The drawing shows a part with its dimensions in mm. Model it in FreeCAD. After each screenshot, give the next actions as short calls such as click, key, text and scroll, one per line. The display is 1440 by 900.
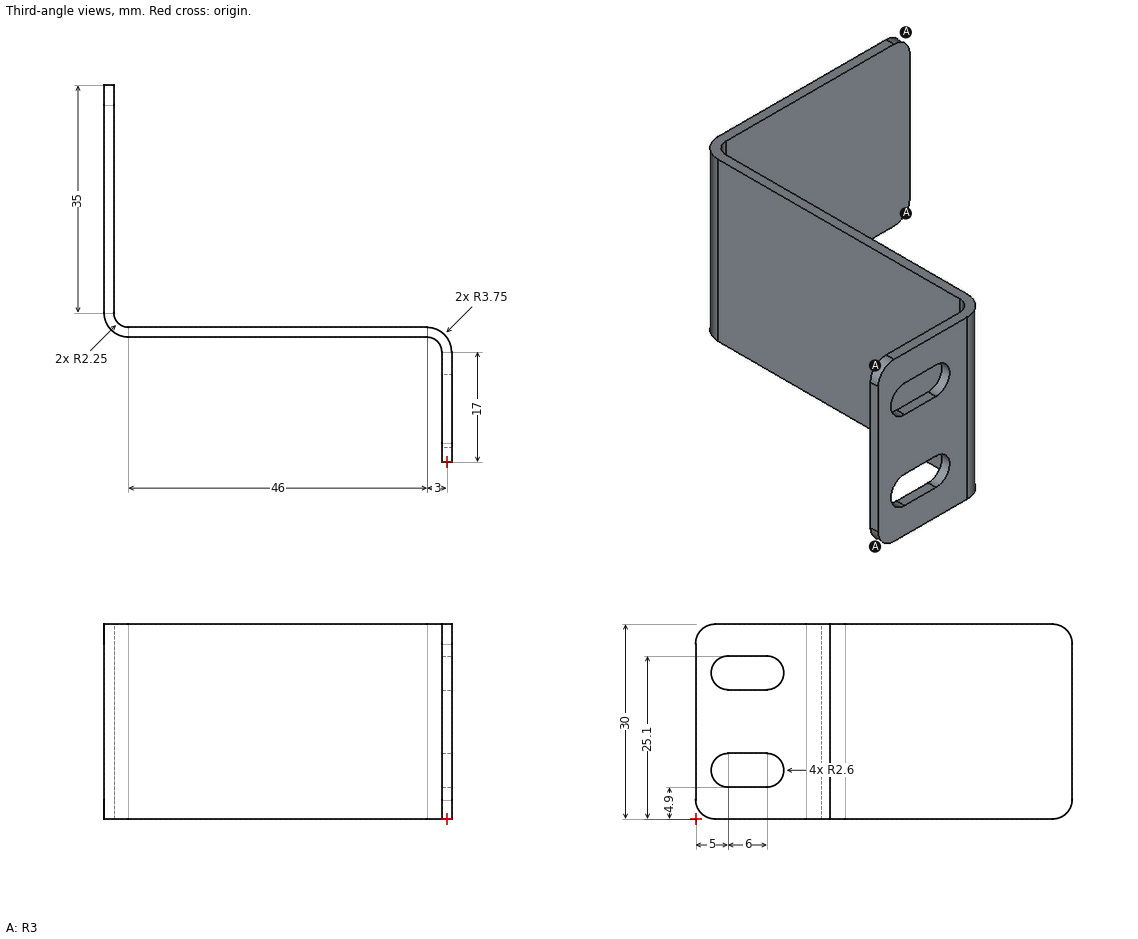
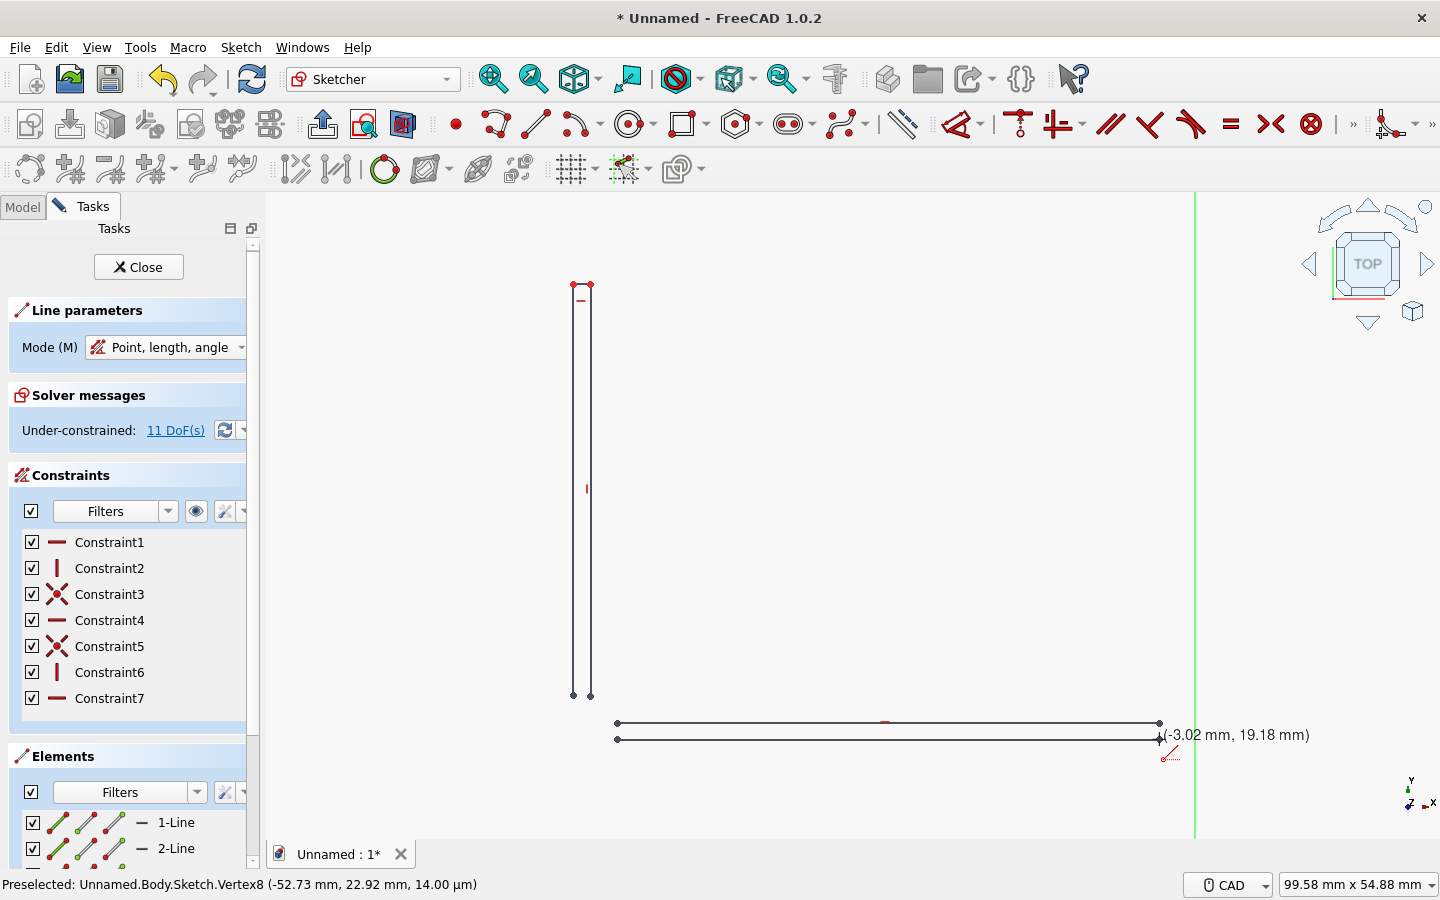
click(496, 124)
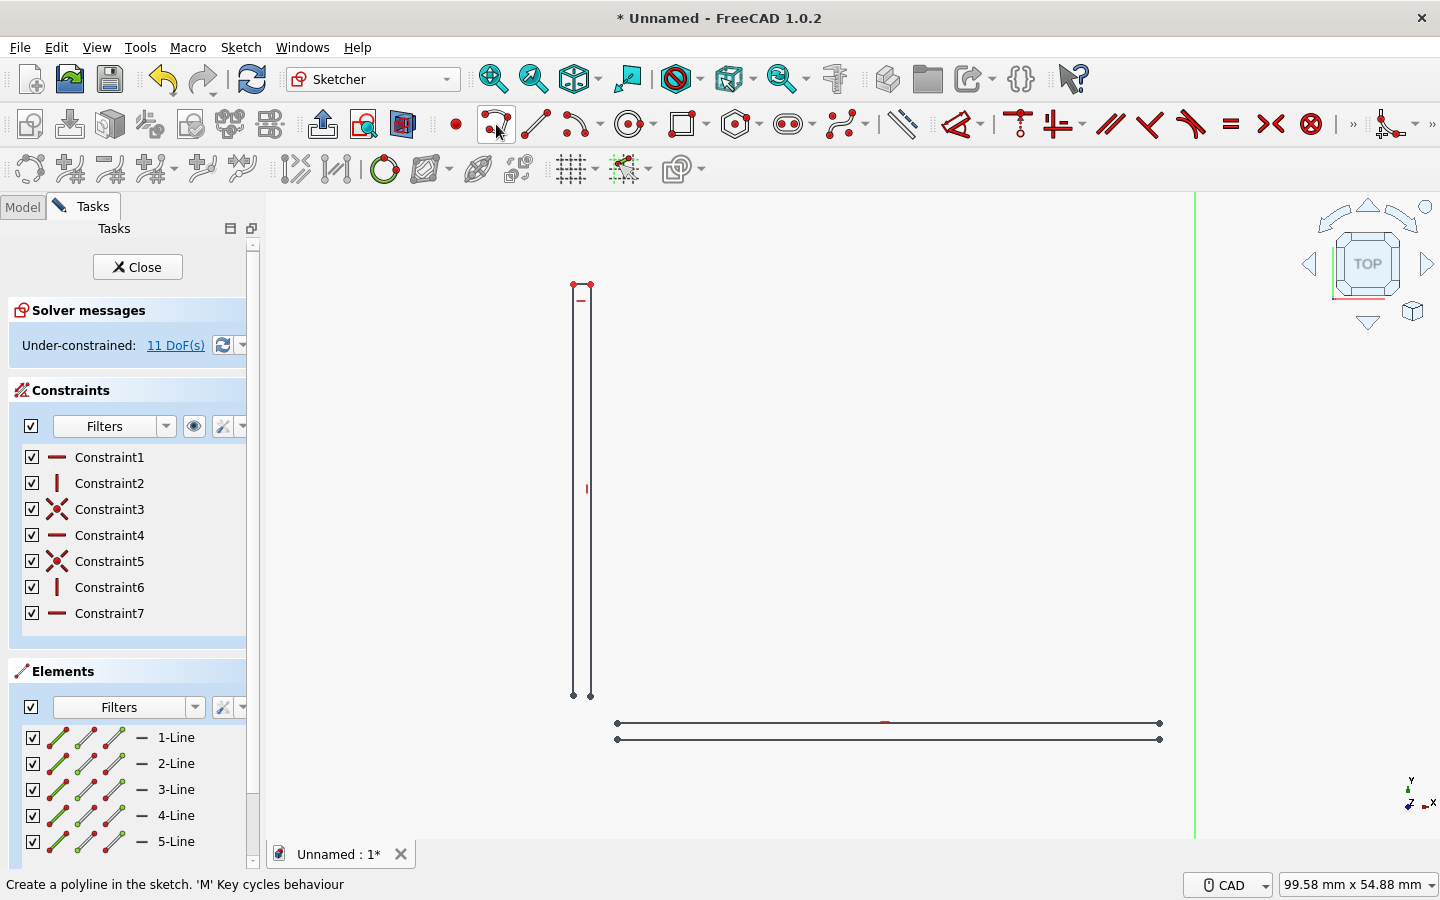
scroll(1186, 766, up, 3)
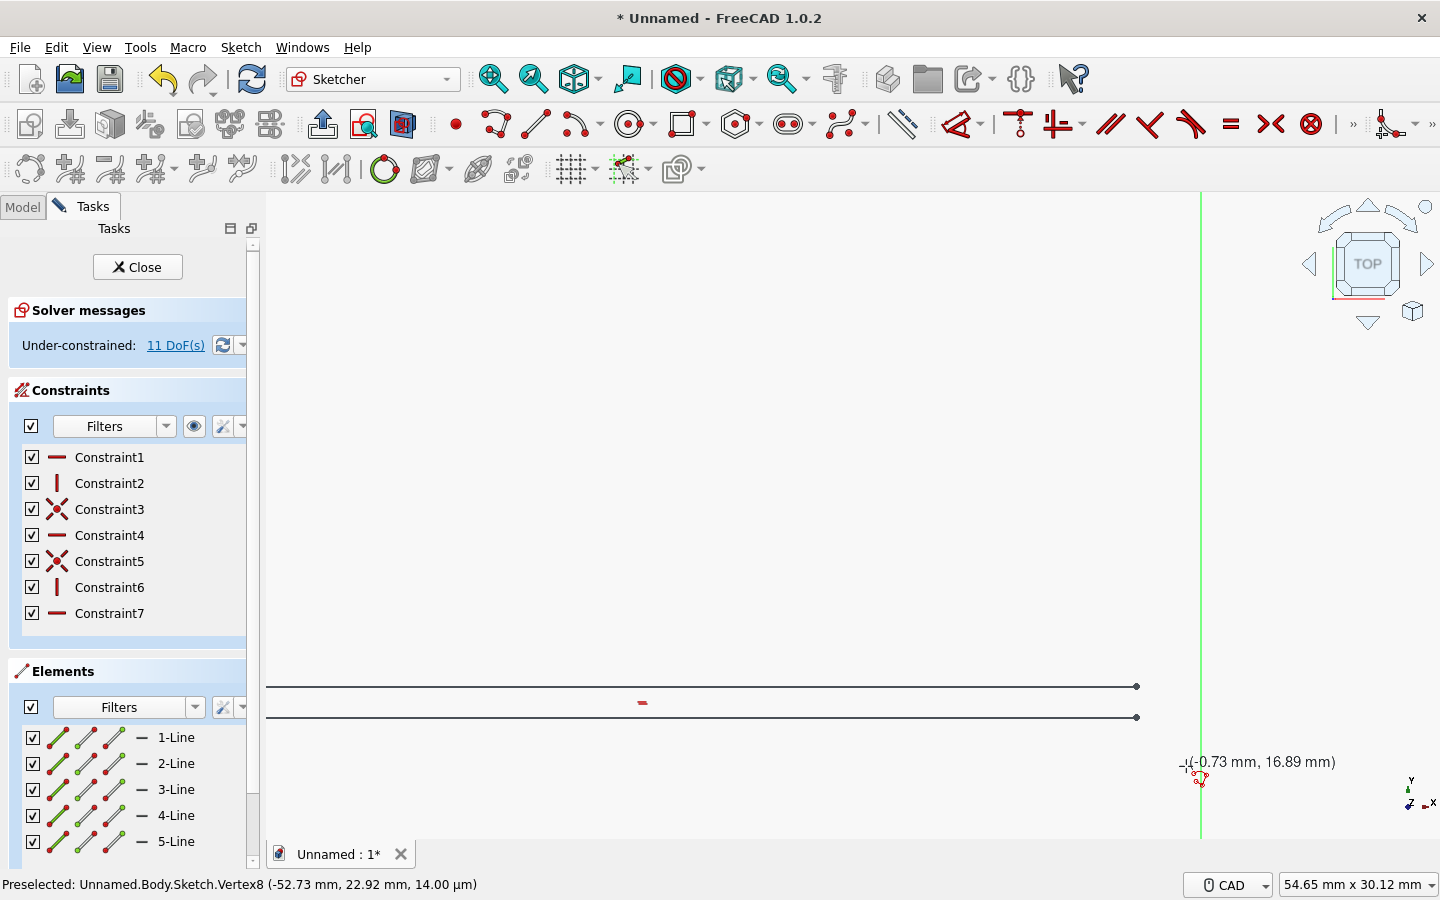
click(1185, 765)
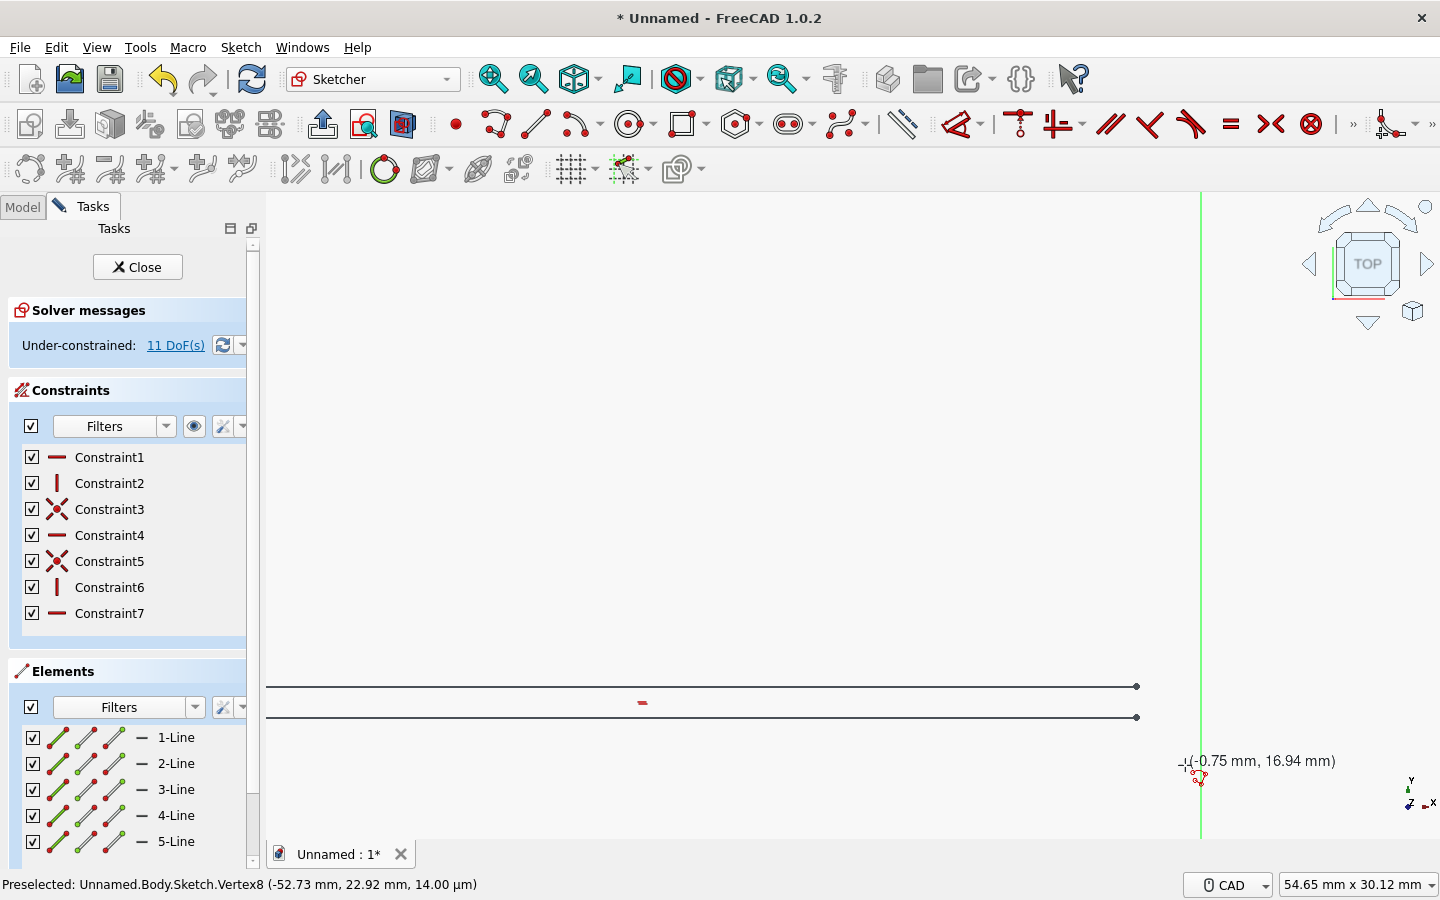
scroll(867, 520, down, 5)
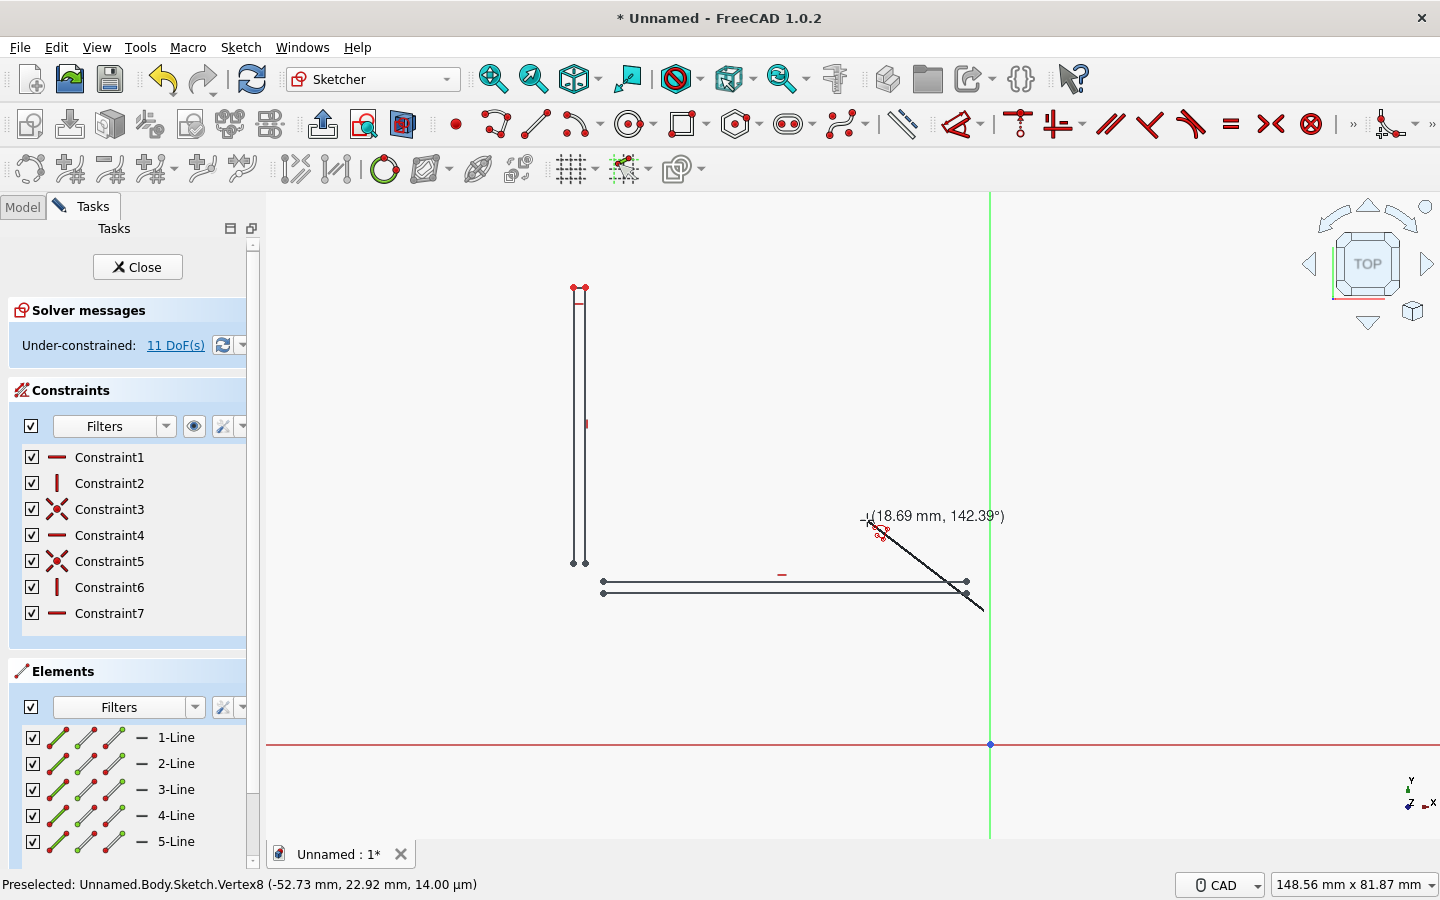
scroll(984, 745, up, 5)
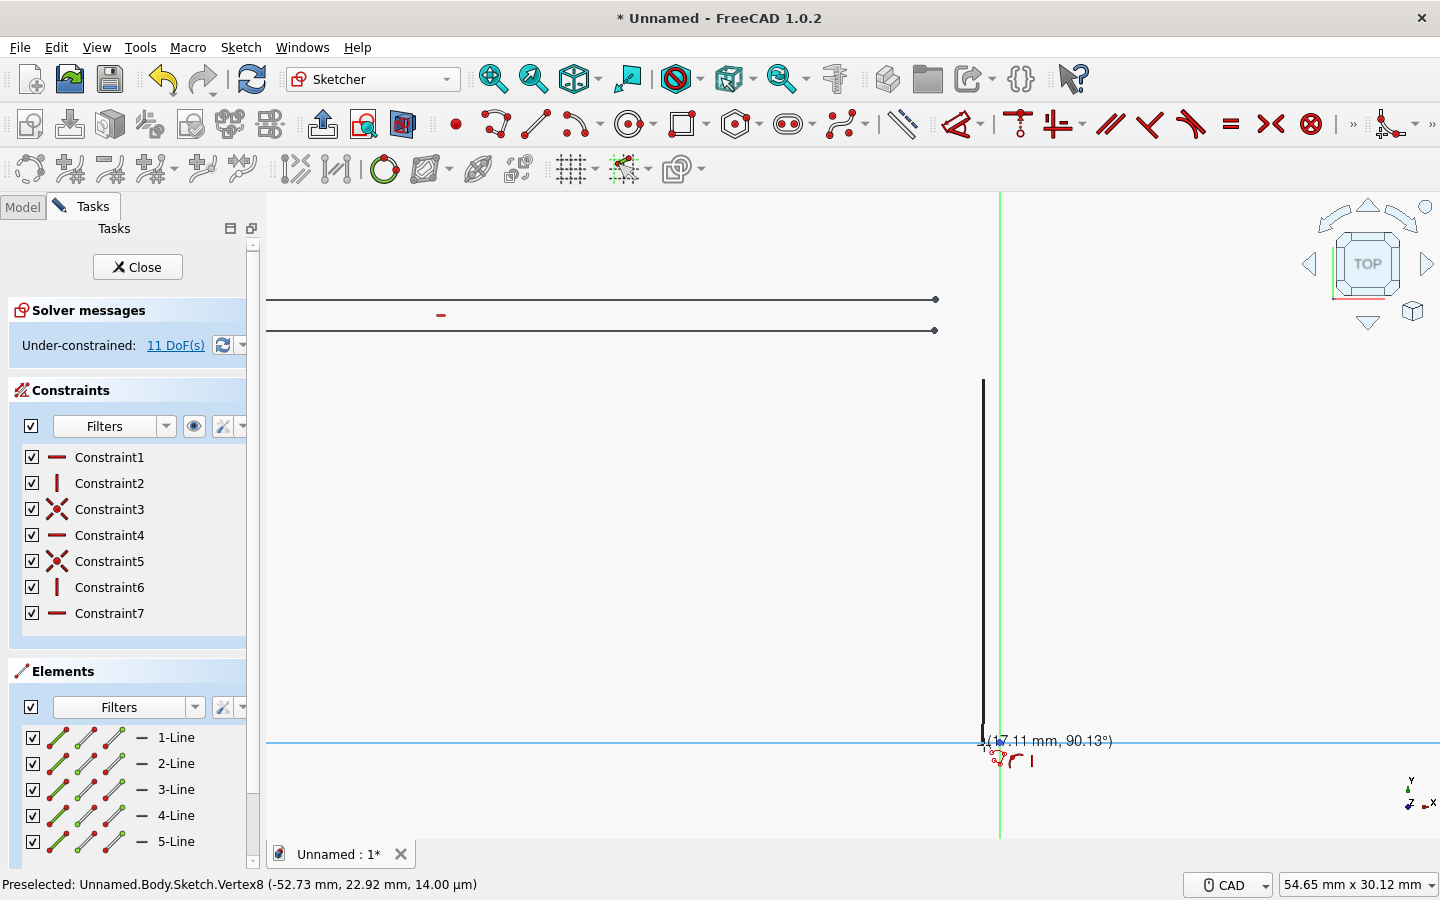
click(984, 743)
click(1016, 734)
click(1016, 378)
right_click(1016, 378)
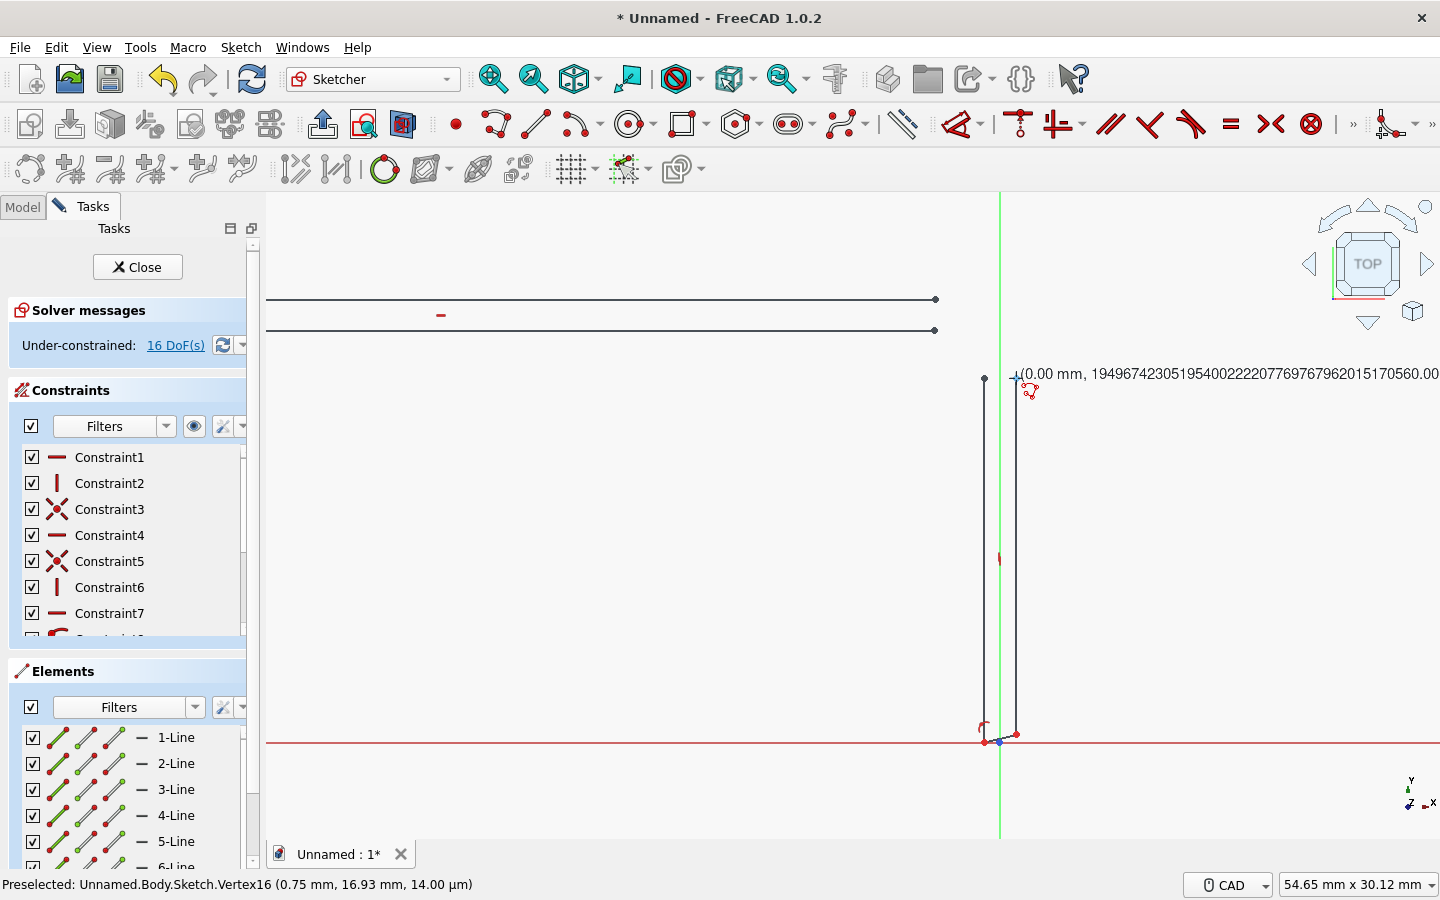
key(g)
key(3)
key(a)